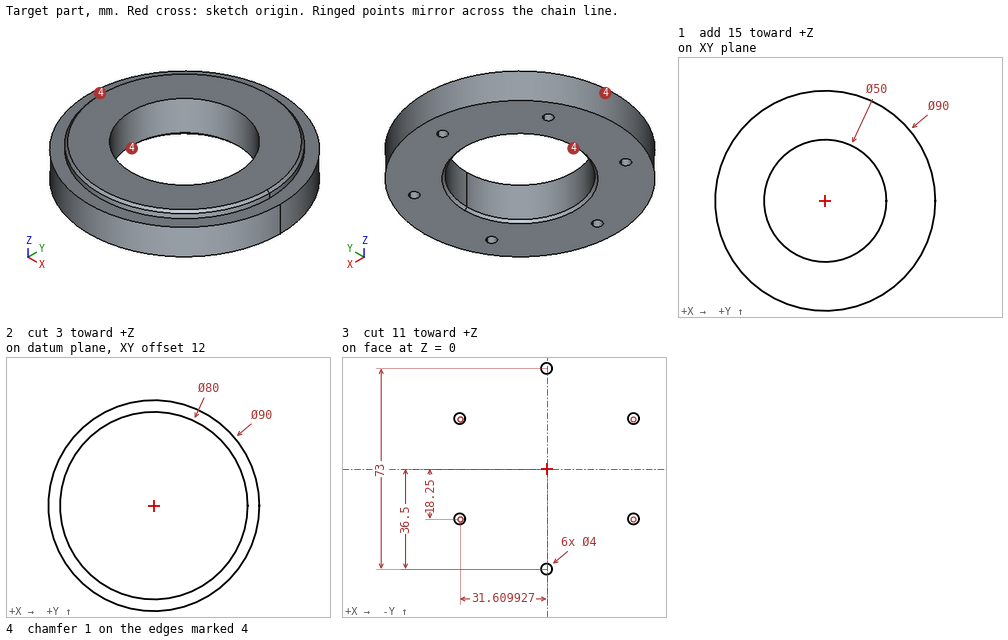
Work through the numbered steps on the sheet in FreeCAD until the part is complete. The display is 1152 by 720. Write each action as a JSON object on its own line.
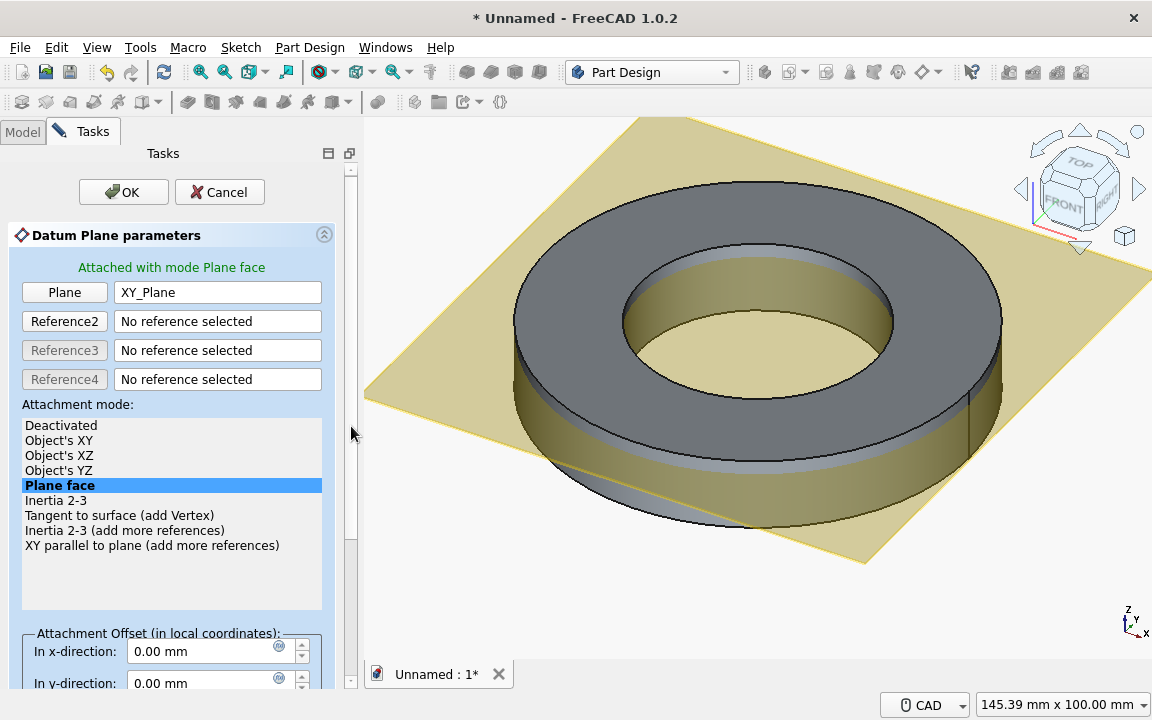
{"action": "left_click", "coordinate": [124, 192]}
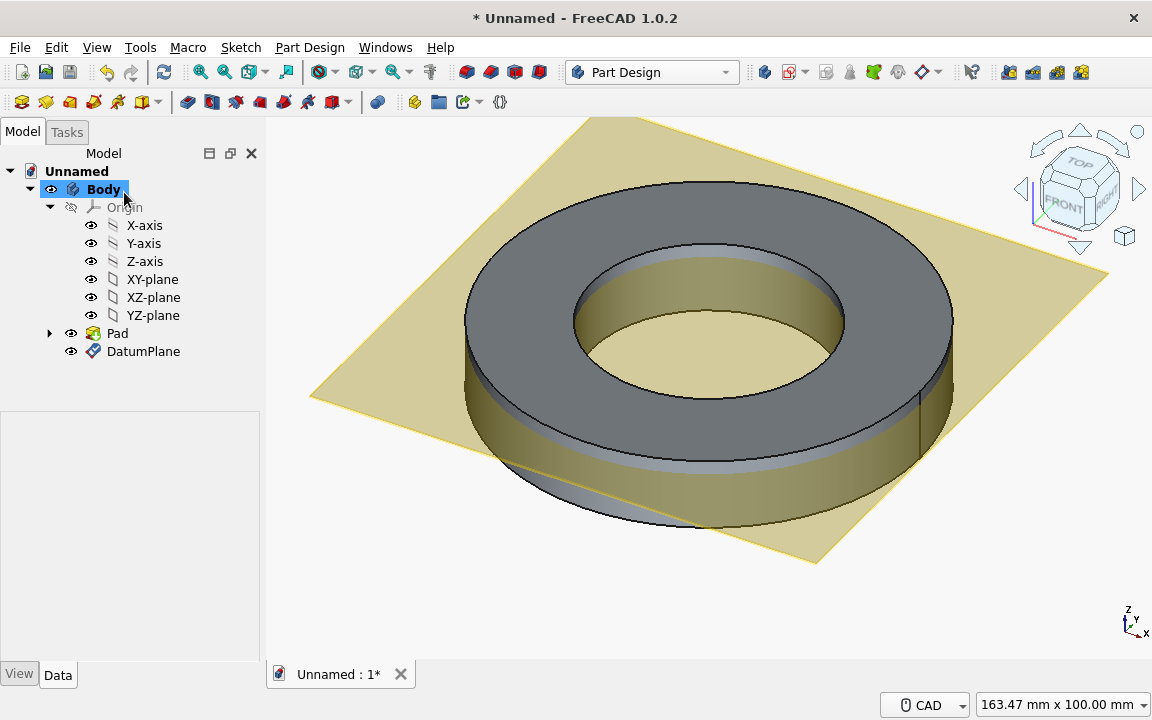
{"action": "left_click", "coordinate": [116, 351]}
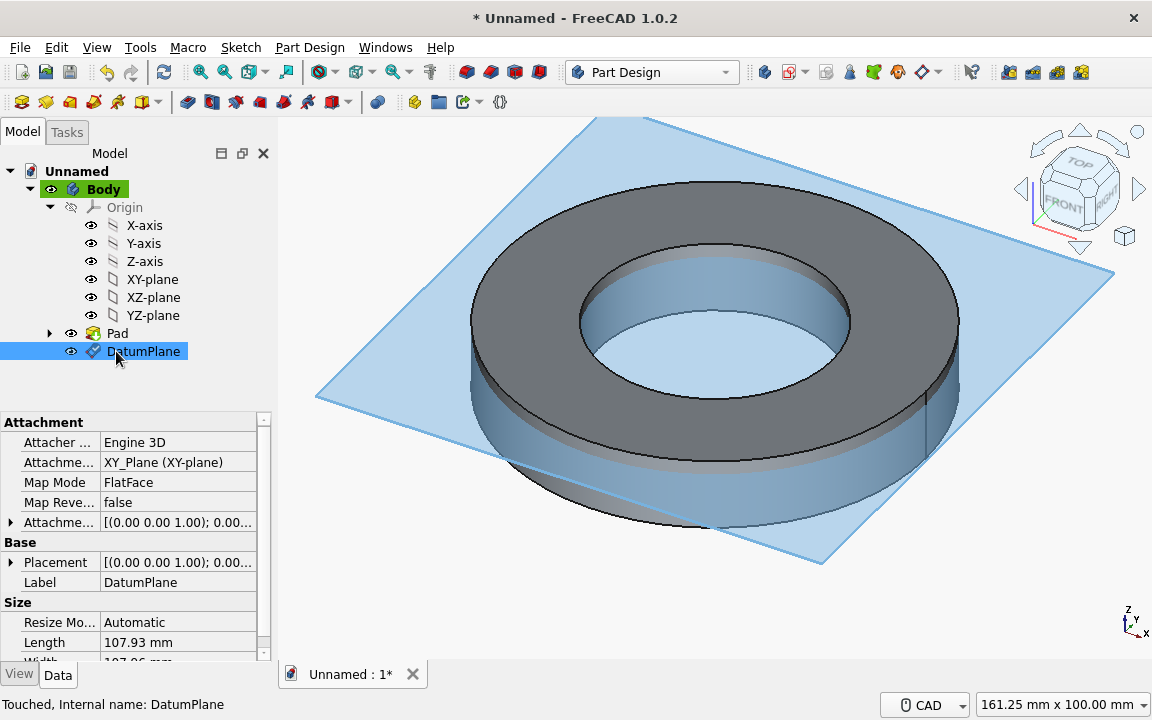
{"action": "left_click", "coordinate": [790, 72]}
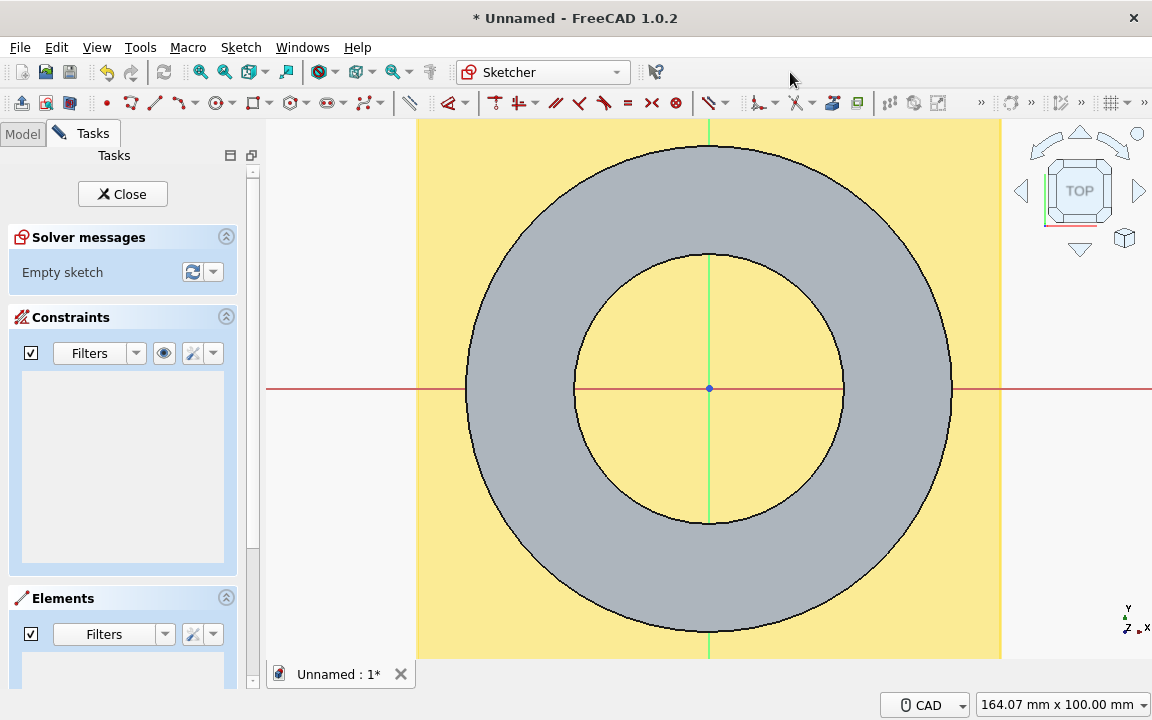
{"action": "left_click", "coordinate": [70, 104]}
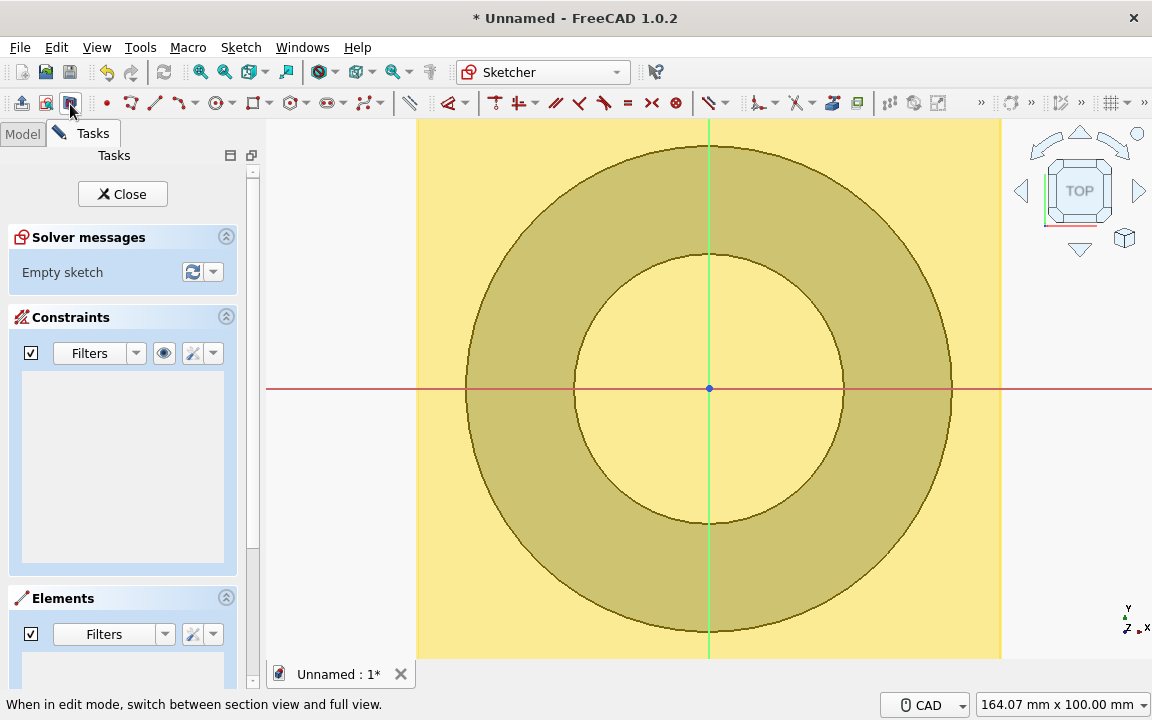
{"action": "scroll", "coordinate": [501, 389], "scroll_direction": "down", "scroll_amount": 2}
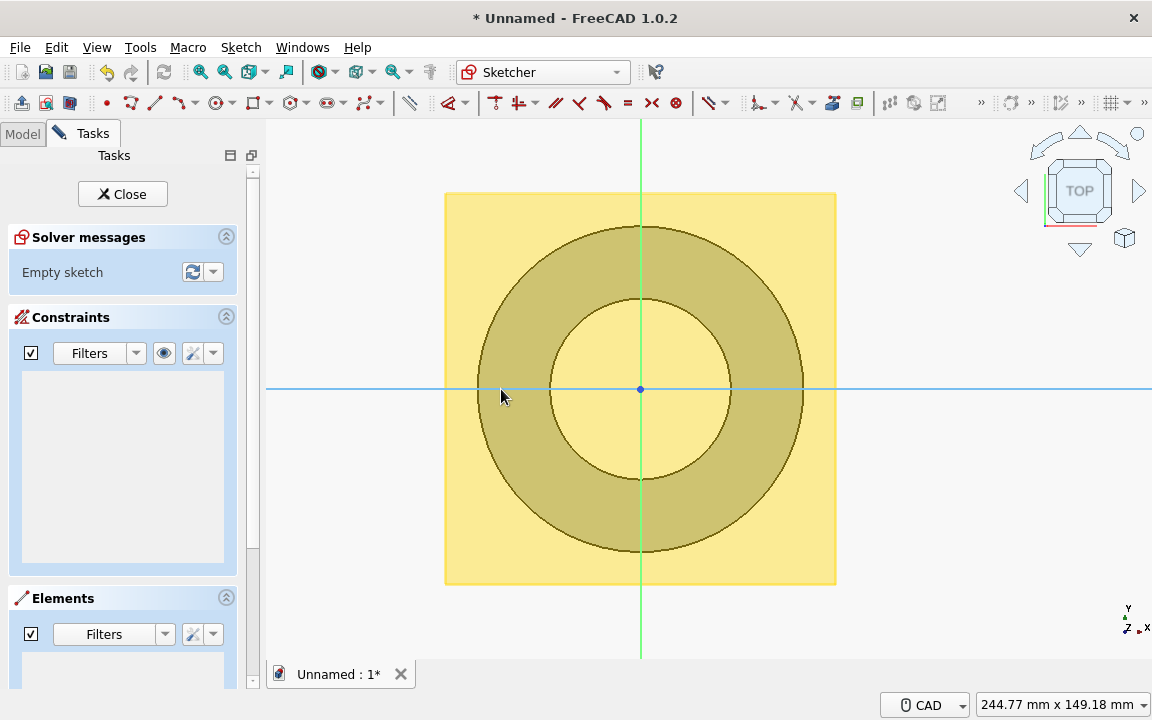
{"action": "left_click", "coordinate": [216, 104]}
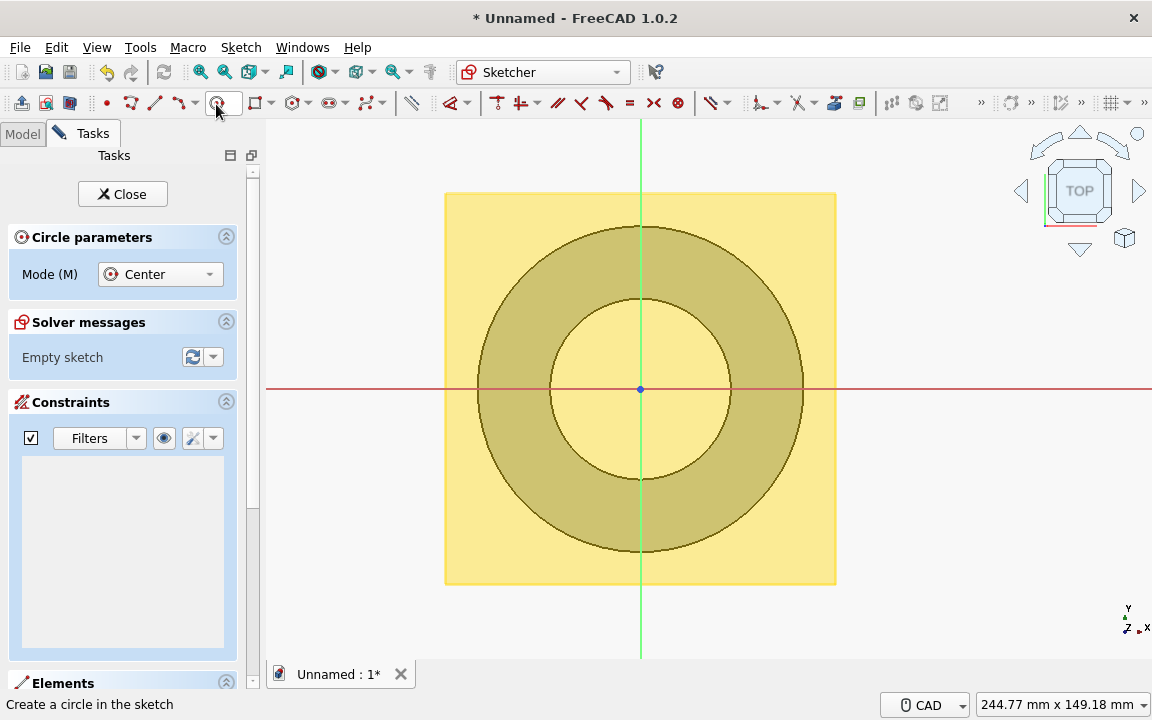
{"action": "left_click", "coordinate": [641, 389]}
{"action": "left_click", "coordinate": [756, 274]}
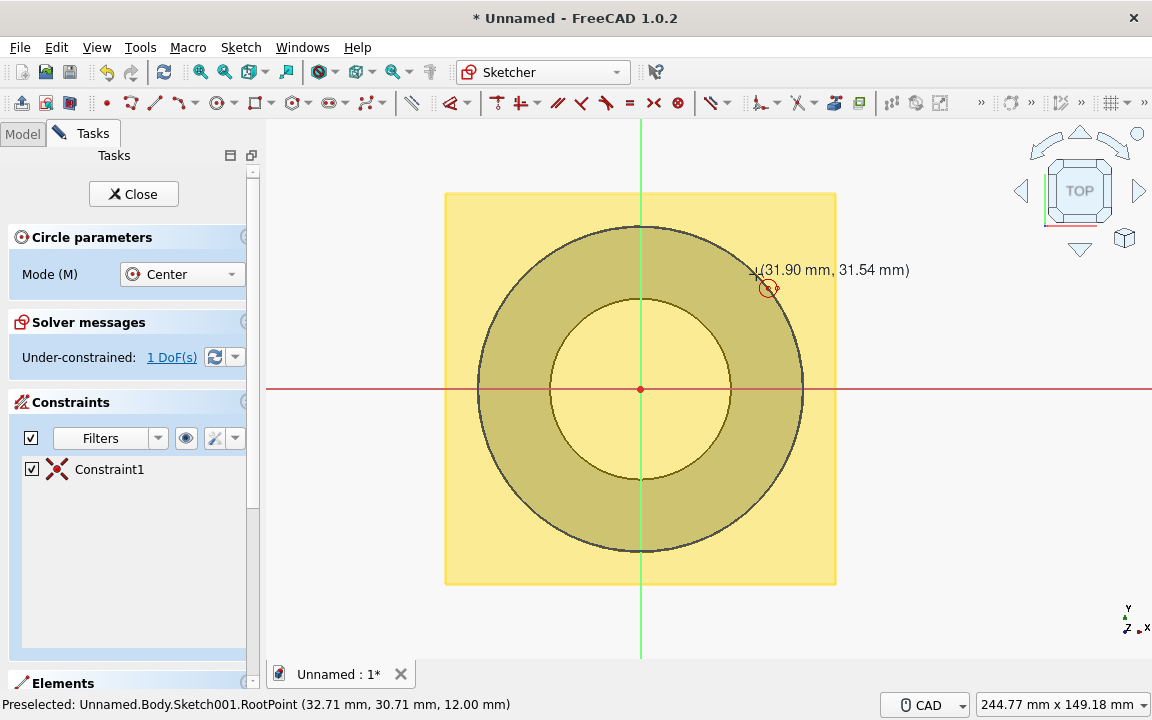
{"action": "left_click", "coordinate": [641, 389]}
{"action": "left_click", "coordinate": [743, 287]}
{"action": "key", "text": "Escape"}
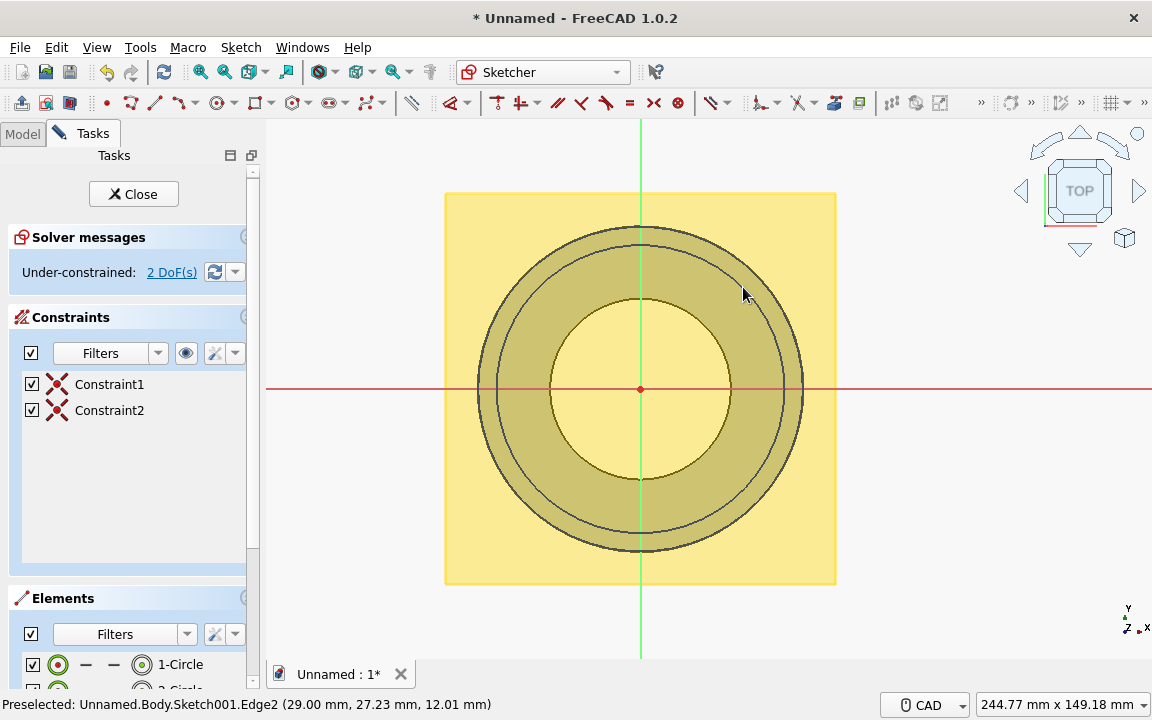
{"action": "left_click", "coordinate": [450, 104]}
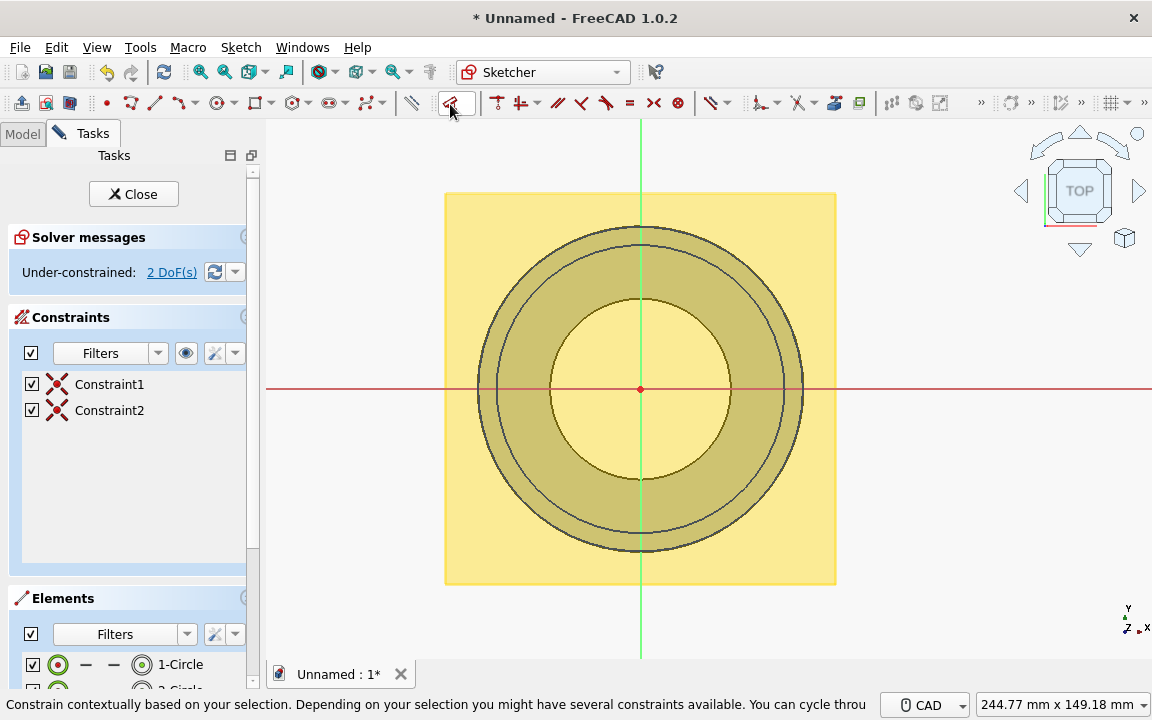
{"action": "left_click", "coordinate": [755, 274]}
{"action": "left_click", "coordinate": [778, 251]}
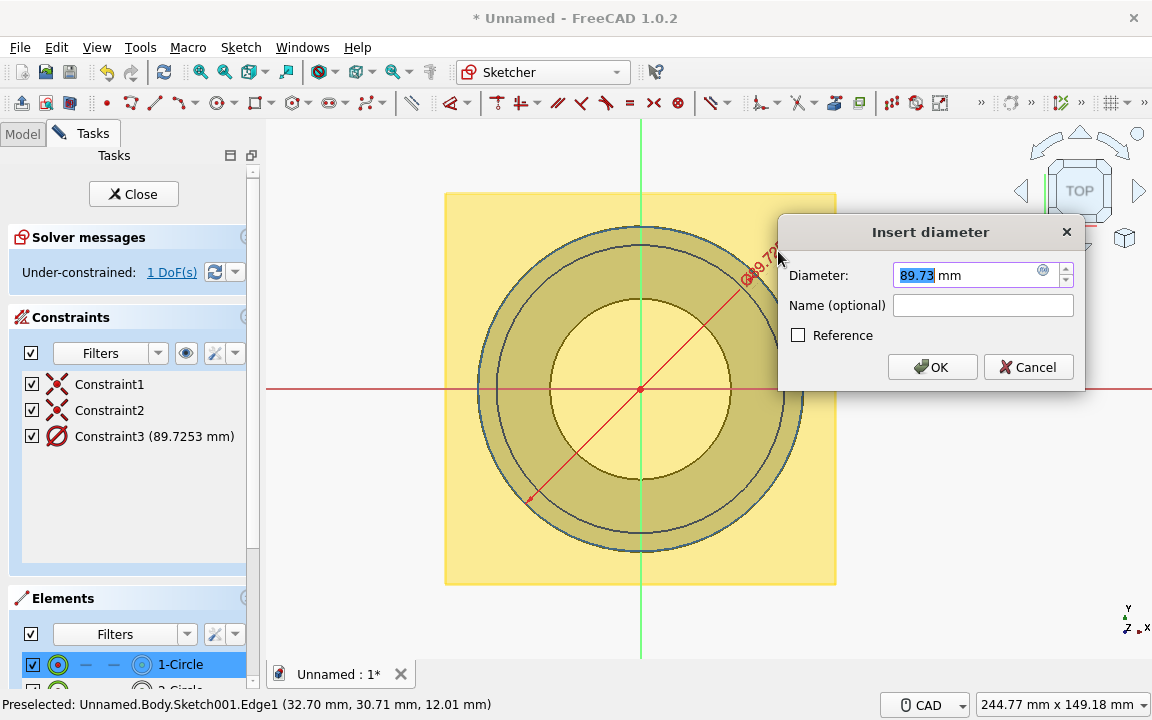
{"action": "type", "text": "90"}
{"action": "key", "text": "Return"}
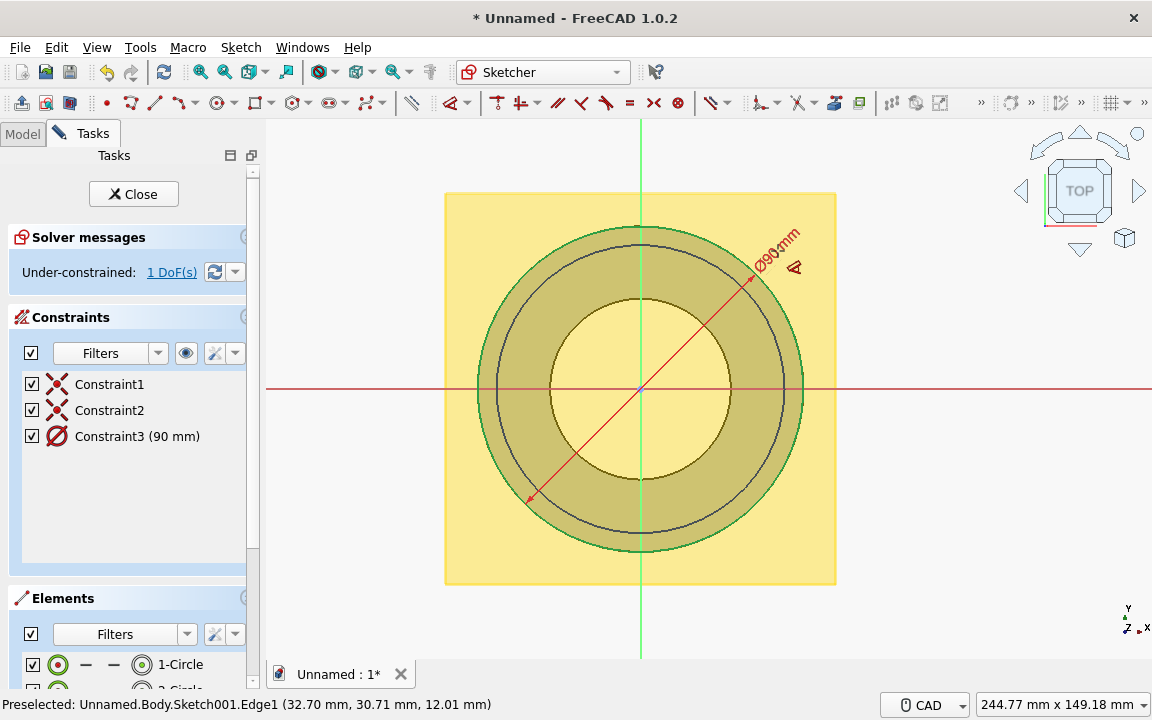
{"action": "left_click", "coordinate": [742, 287]}
{"action": "left_click", "coordinate": [809, 339]}